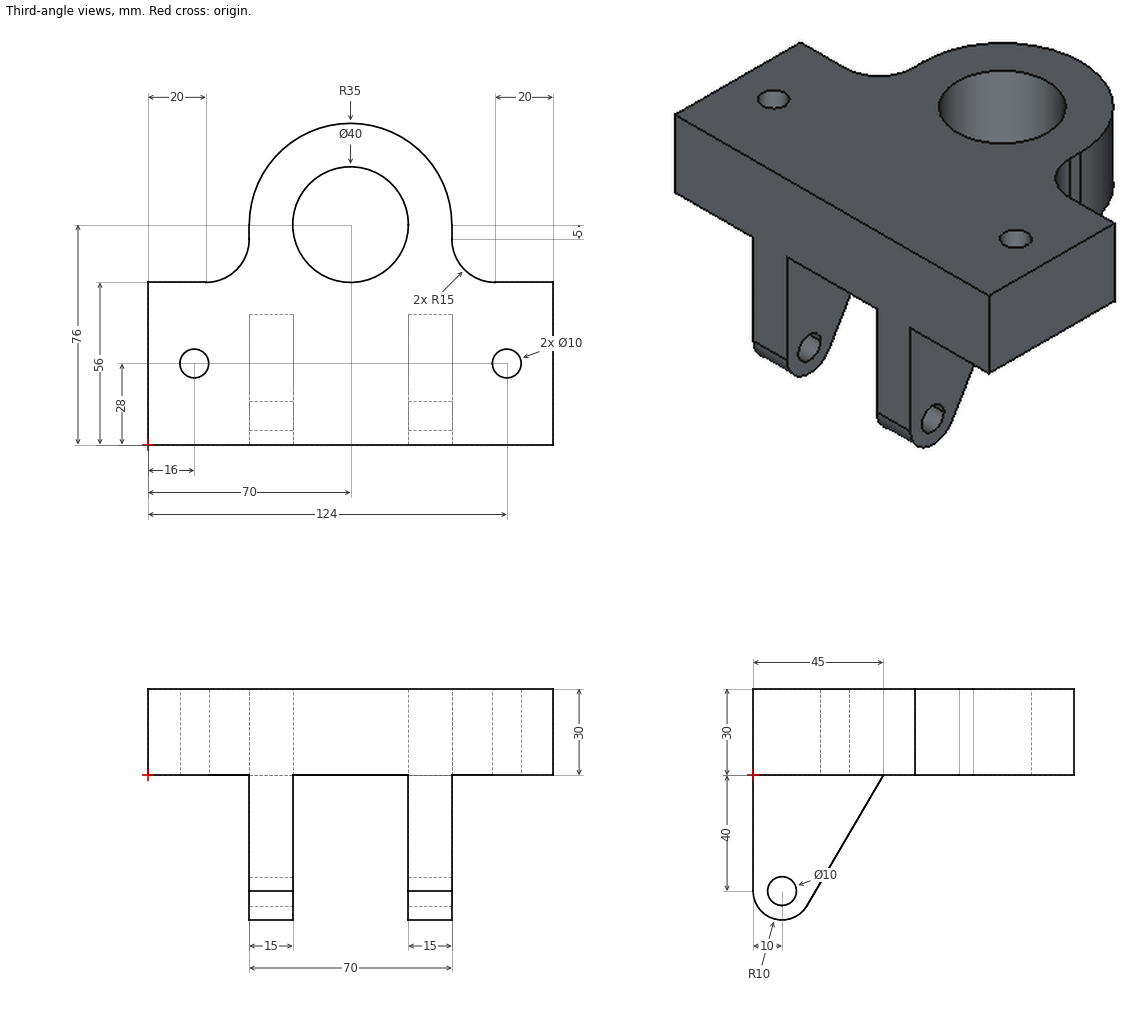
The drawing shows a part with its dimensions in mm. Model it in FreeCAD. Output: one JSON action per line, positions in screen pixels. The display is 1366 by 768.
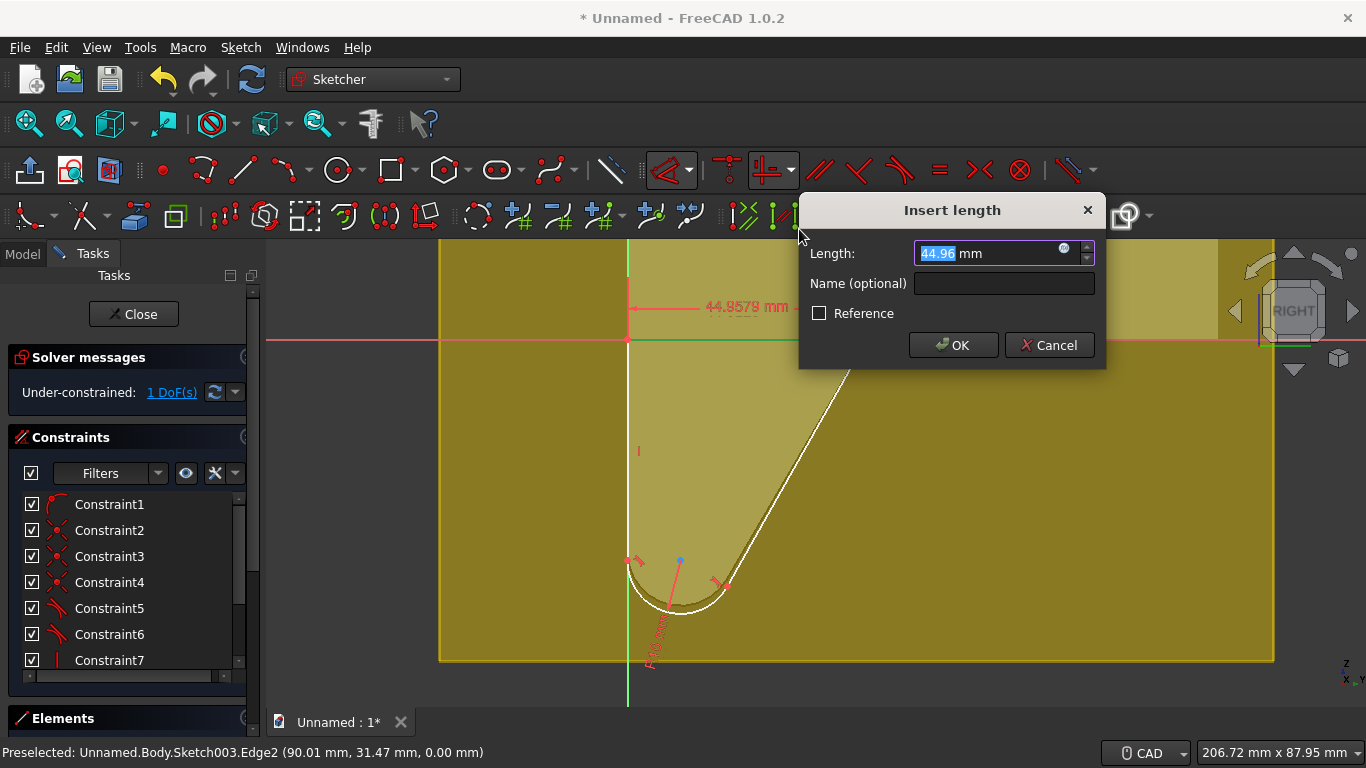
{"action": "type", "text": "45"}
{"action": "key", "text": "Return"}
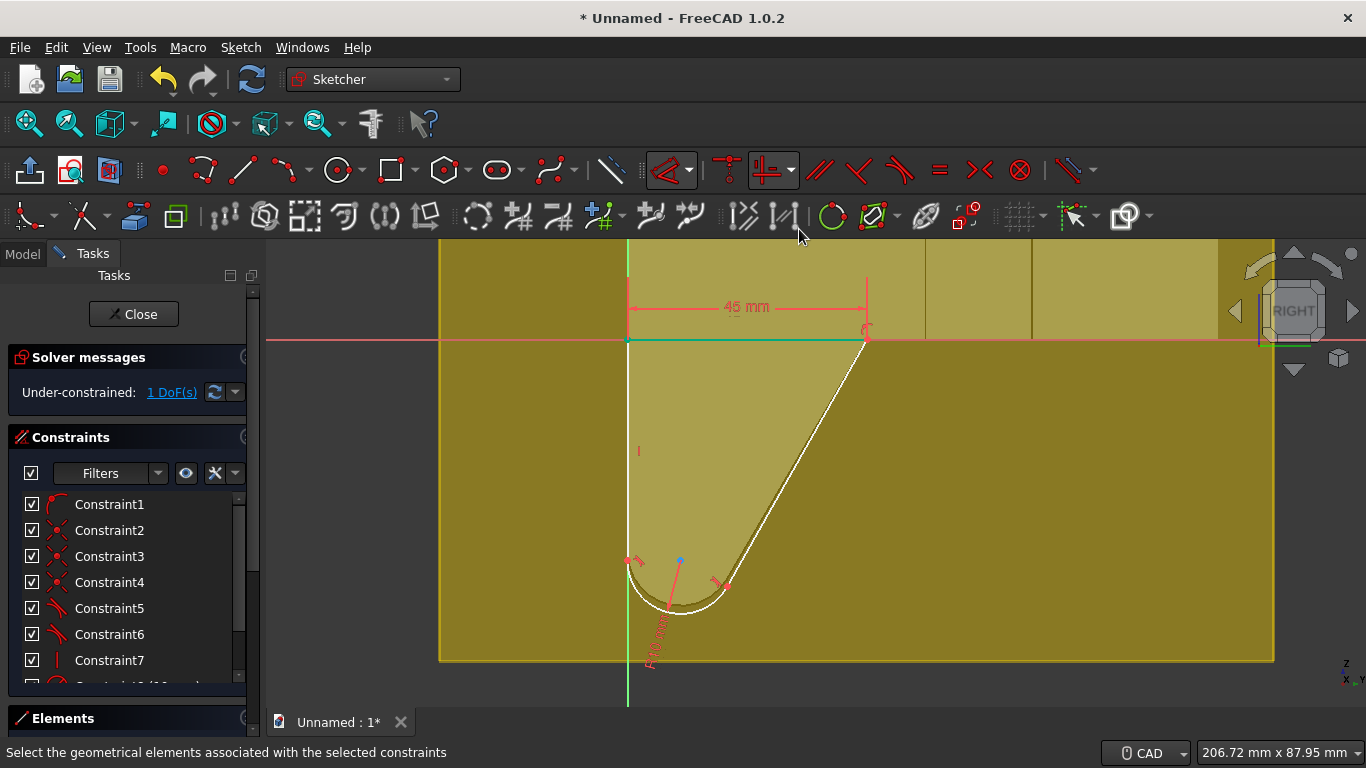
{"action": "left_click", "coordinate": [628, 406]}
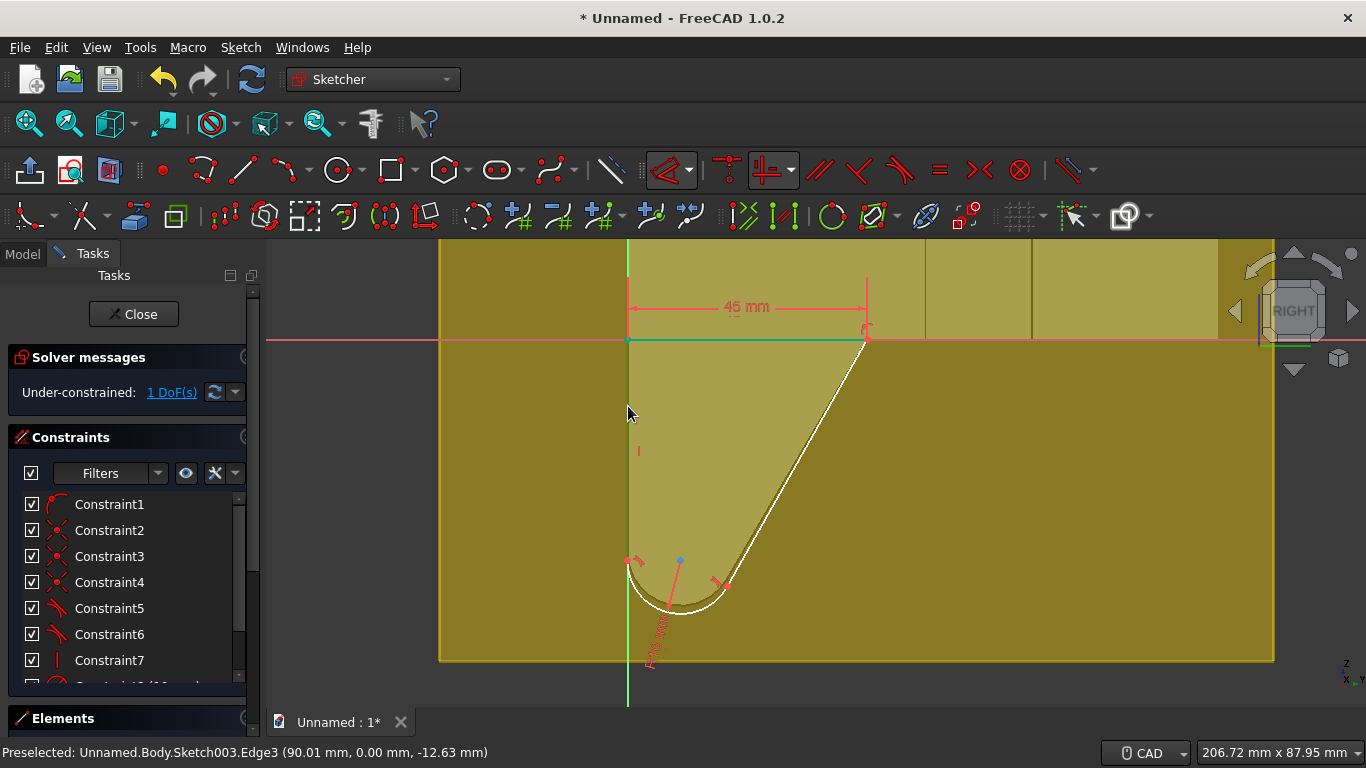
{"action": "left_click", "coordinate": [692, 170]}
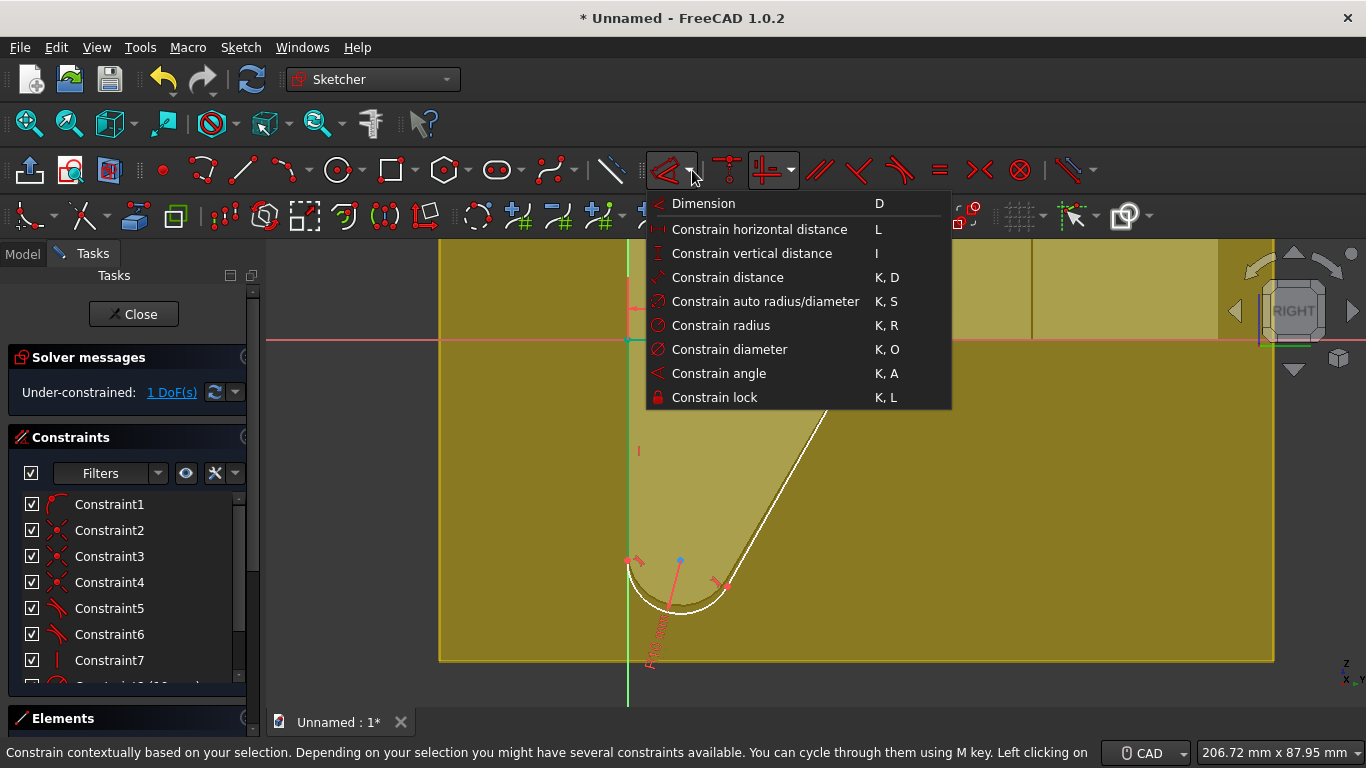
{"action": "left_click", "coordinate": [799, 253]}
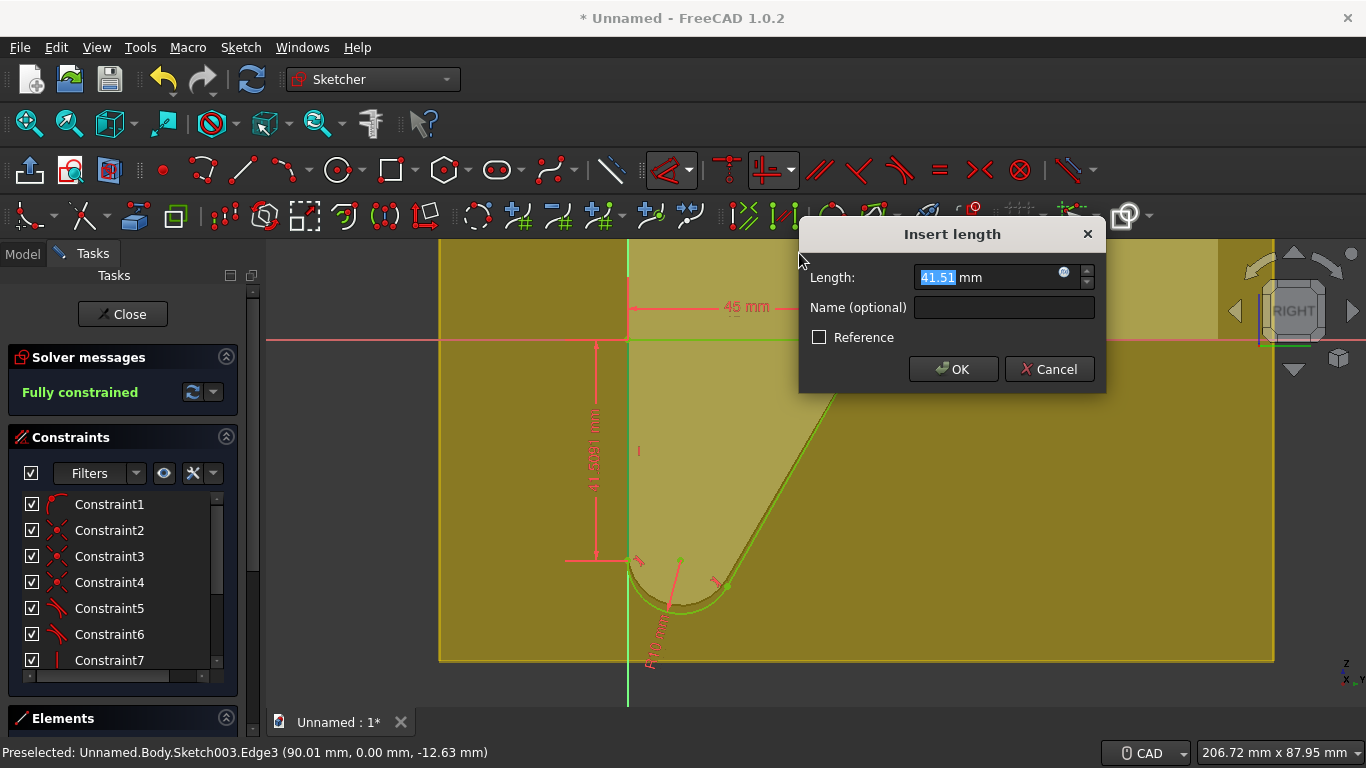
{"action": "type", "text": "40"}
{"action": "key", "text": "Return"}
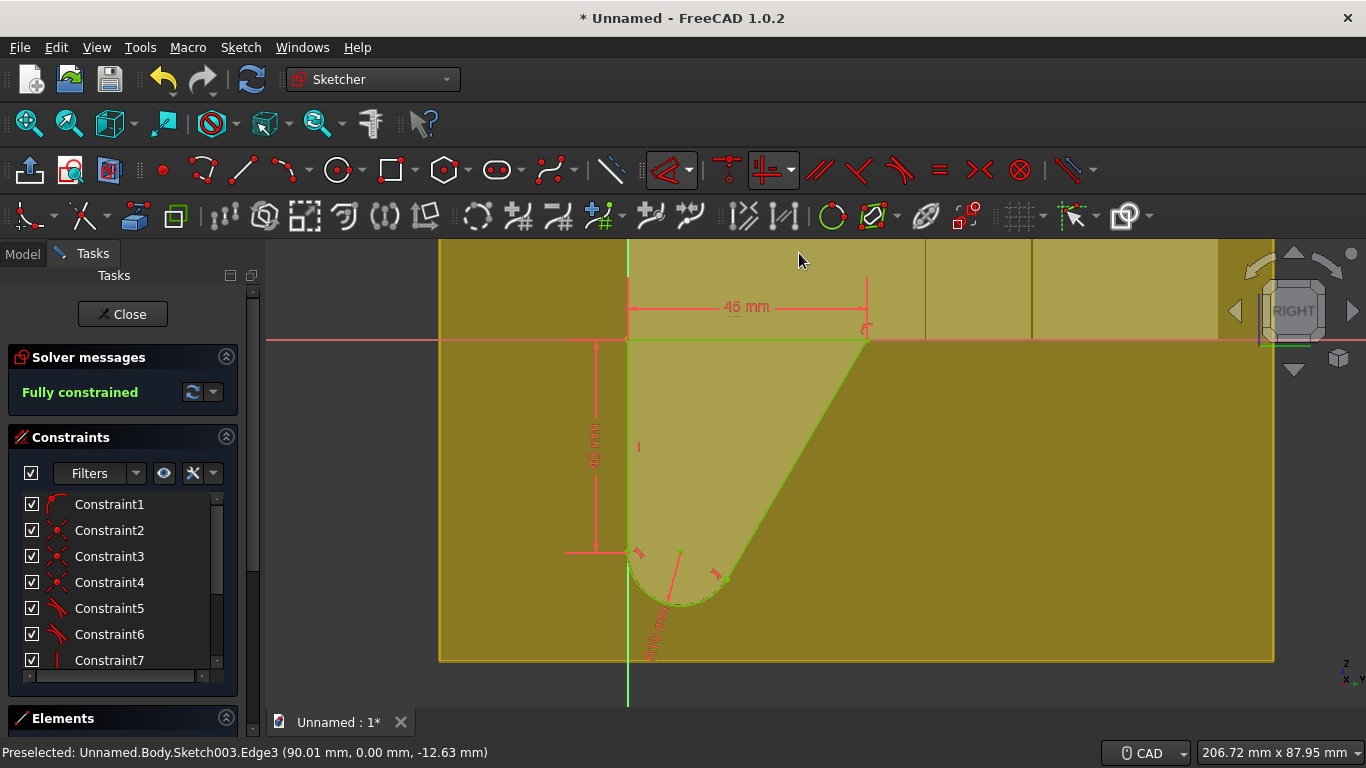
{"action": "left_click", "coordinate": [123, 314]}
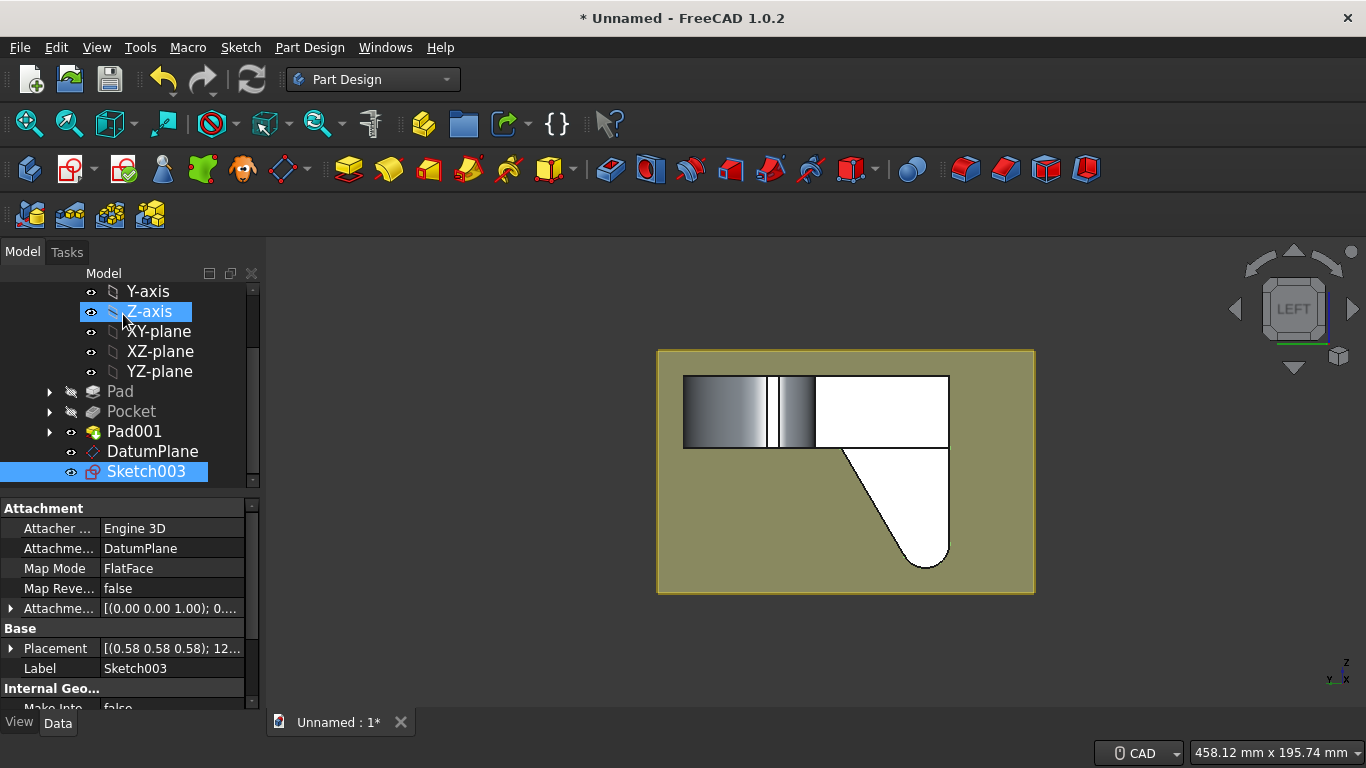
{"action": "left_click", "coordinate": [350, 170]}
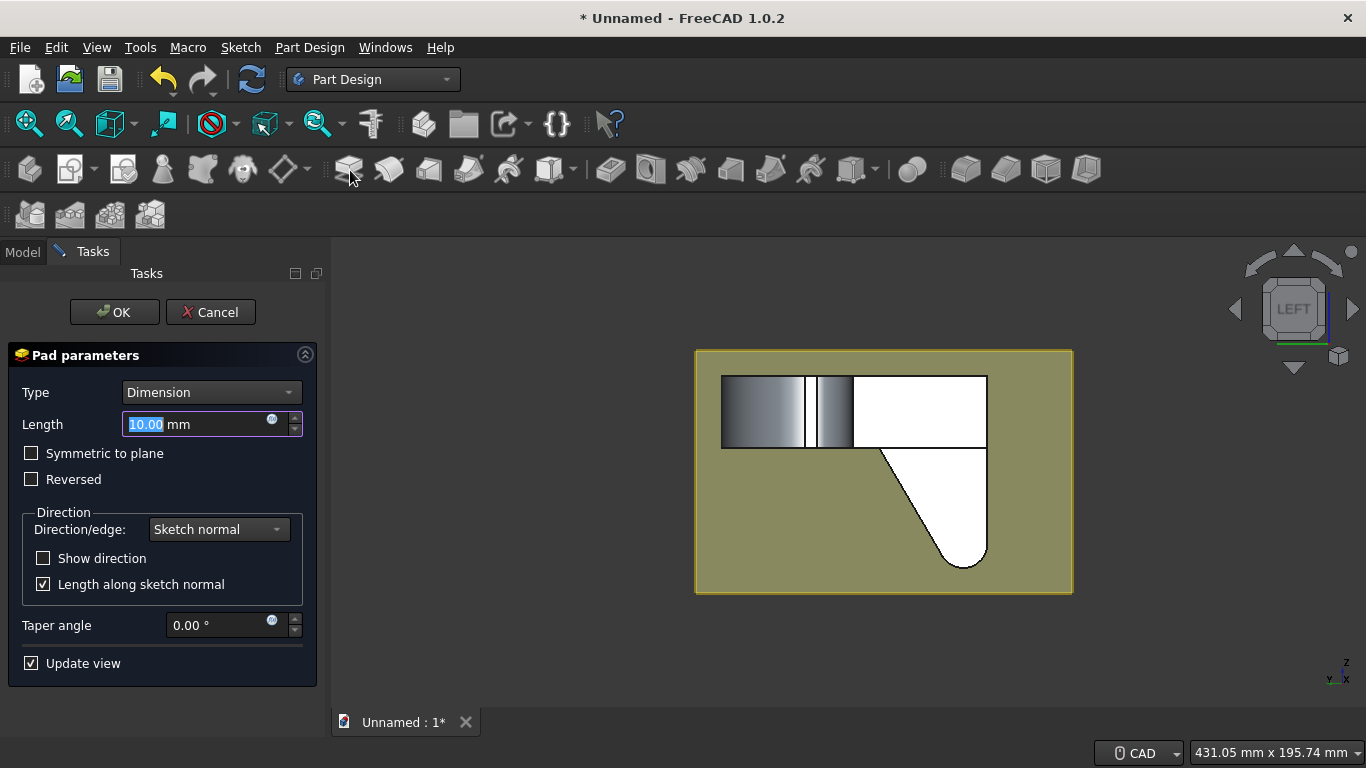
{"action": "type", "text": "15"}
{"action": "key", "text": "Tab"}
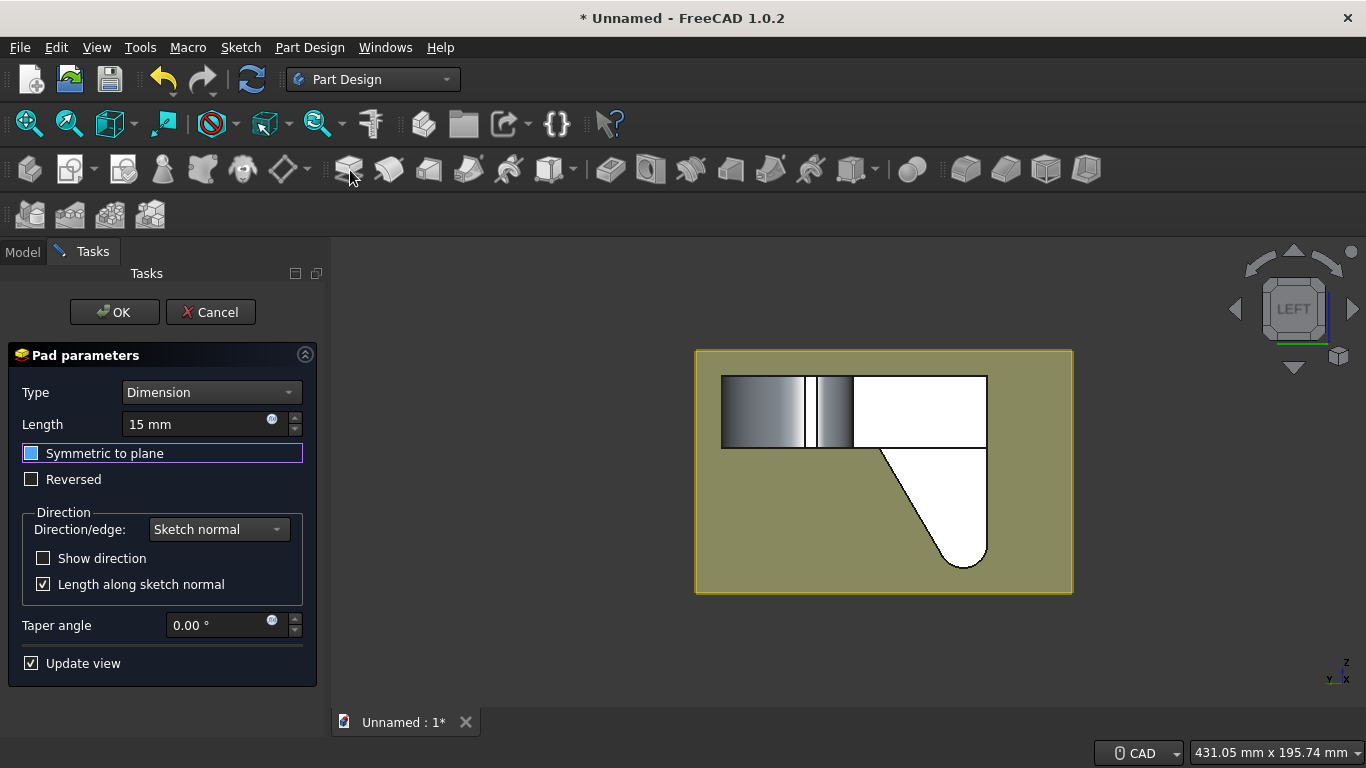
{"action": "left_click", "coordinate": [115, 312]}